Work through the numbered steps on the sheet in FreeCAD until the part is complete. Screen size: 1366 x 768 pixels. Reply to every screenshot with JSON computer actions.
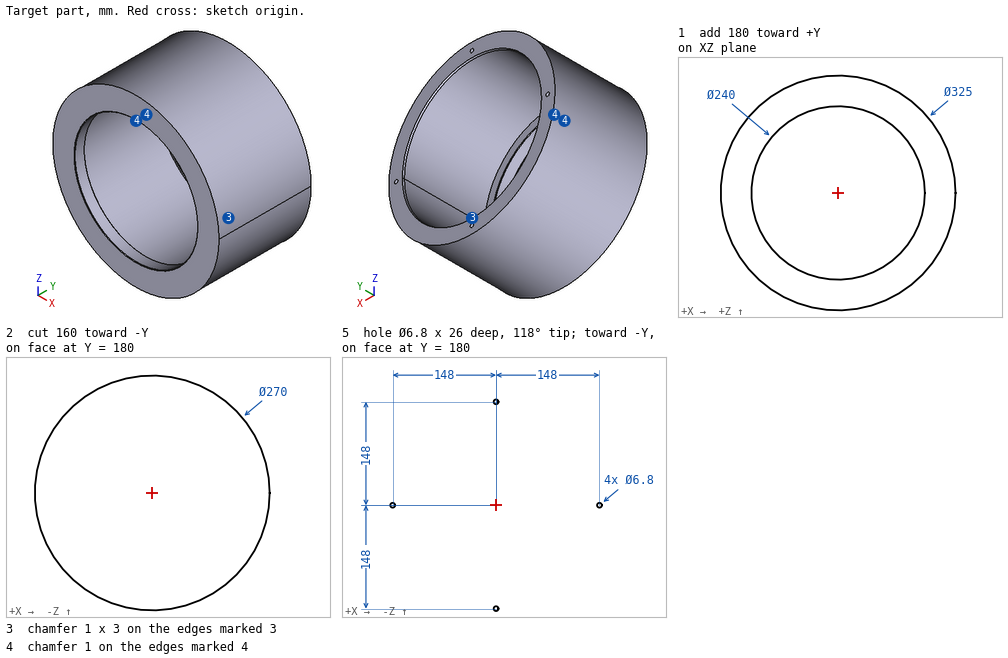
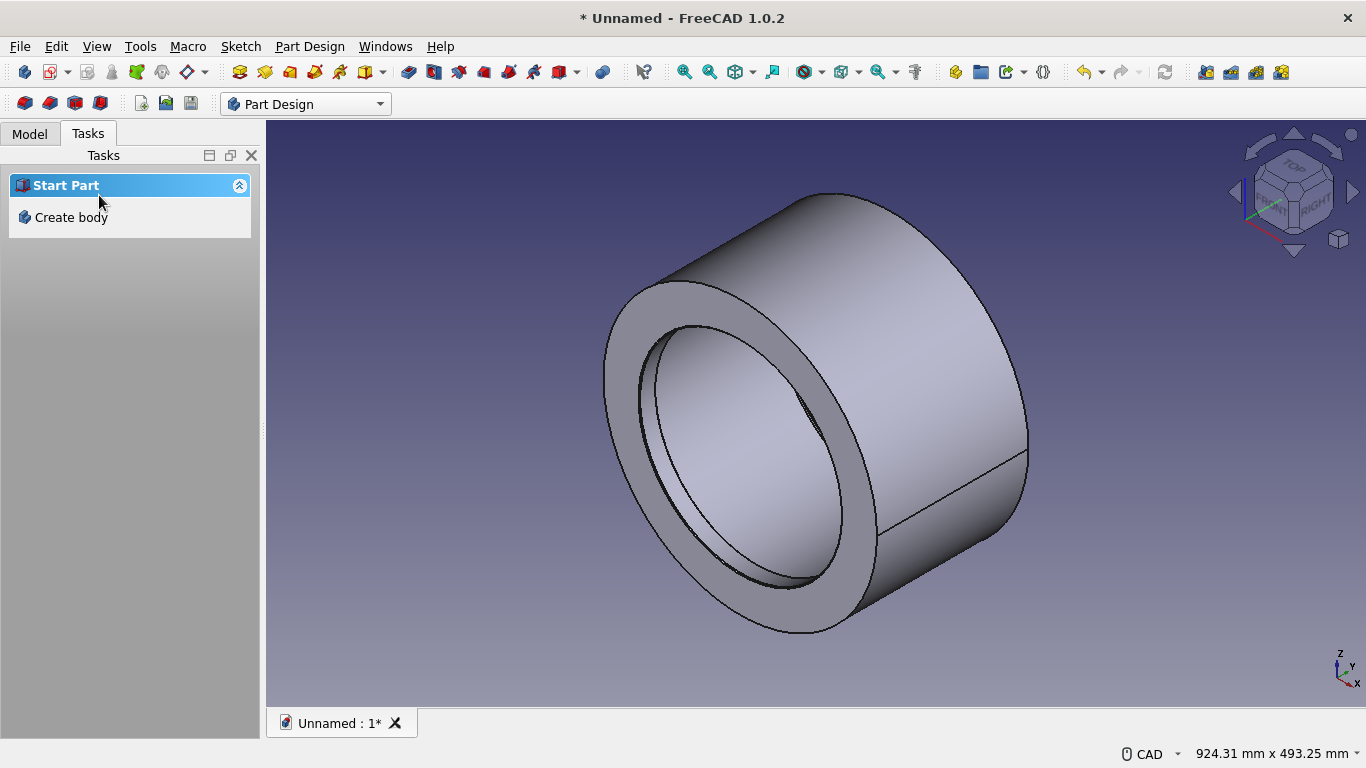
{"action": "key", "text": "4"}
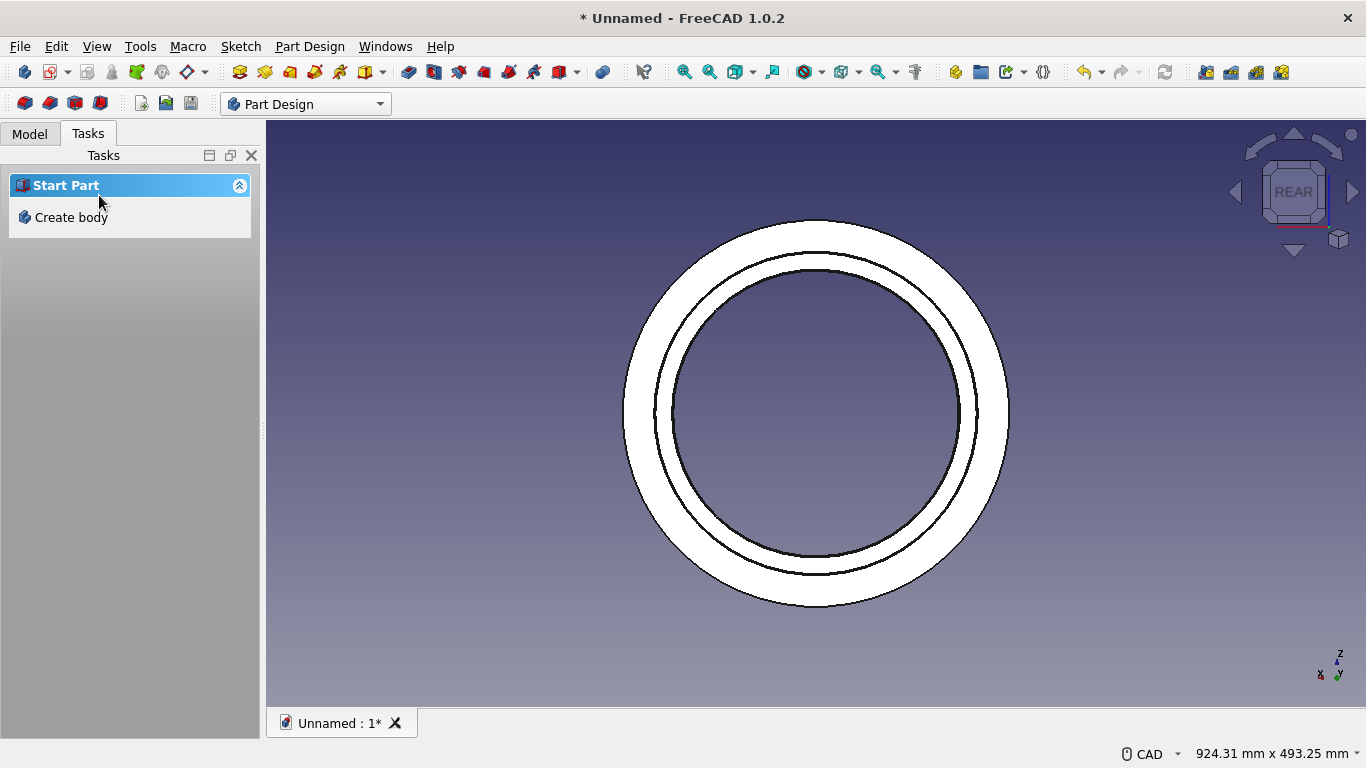
{"action": "left_click", "coordinate": [761, 578]}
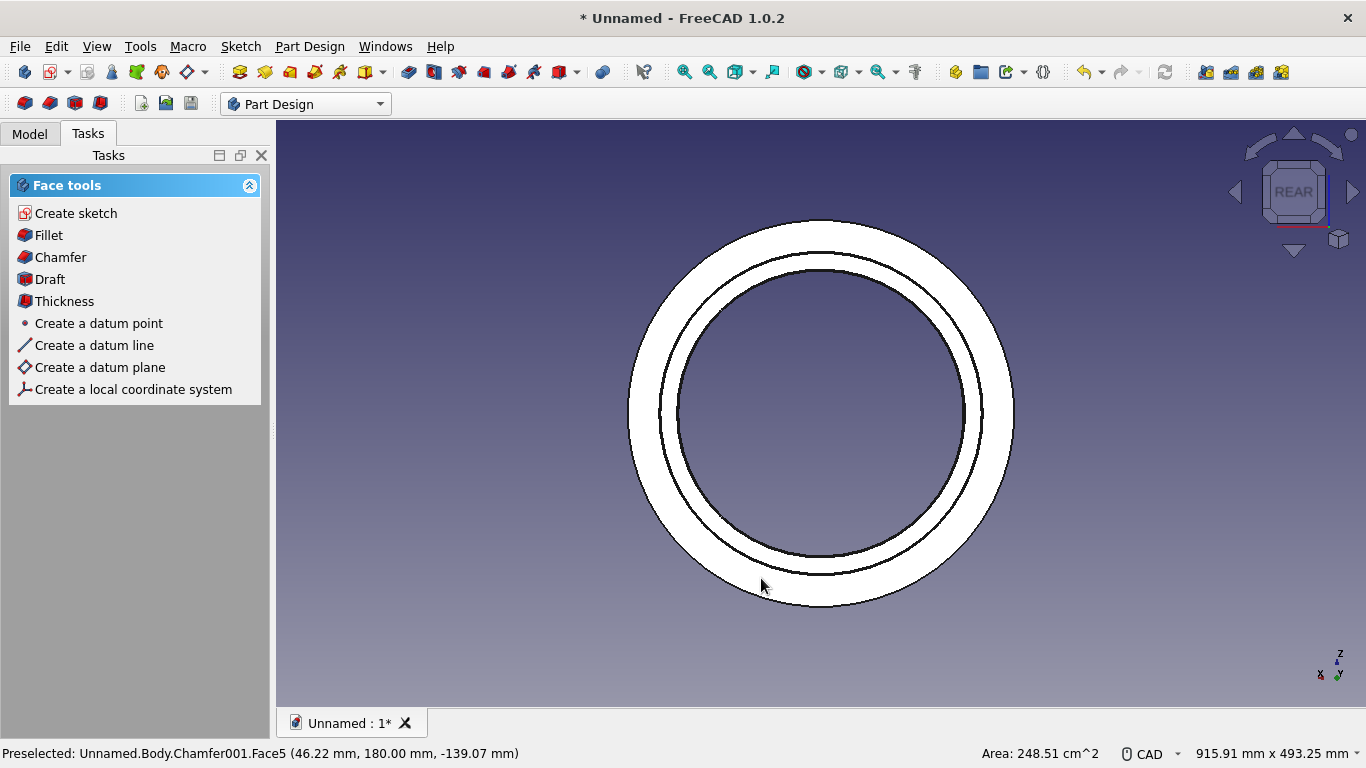
{"action": "left_click", "coordinate": [50, 72]}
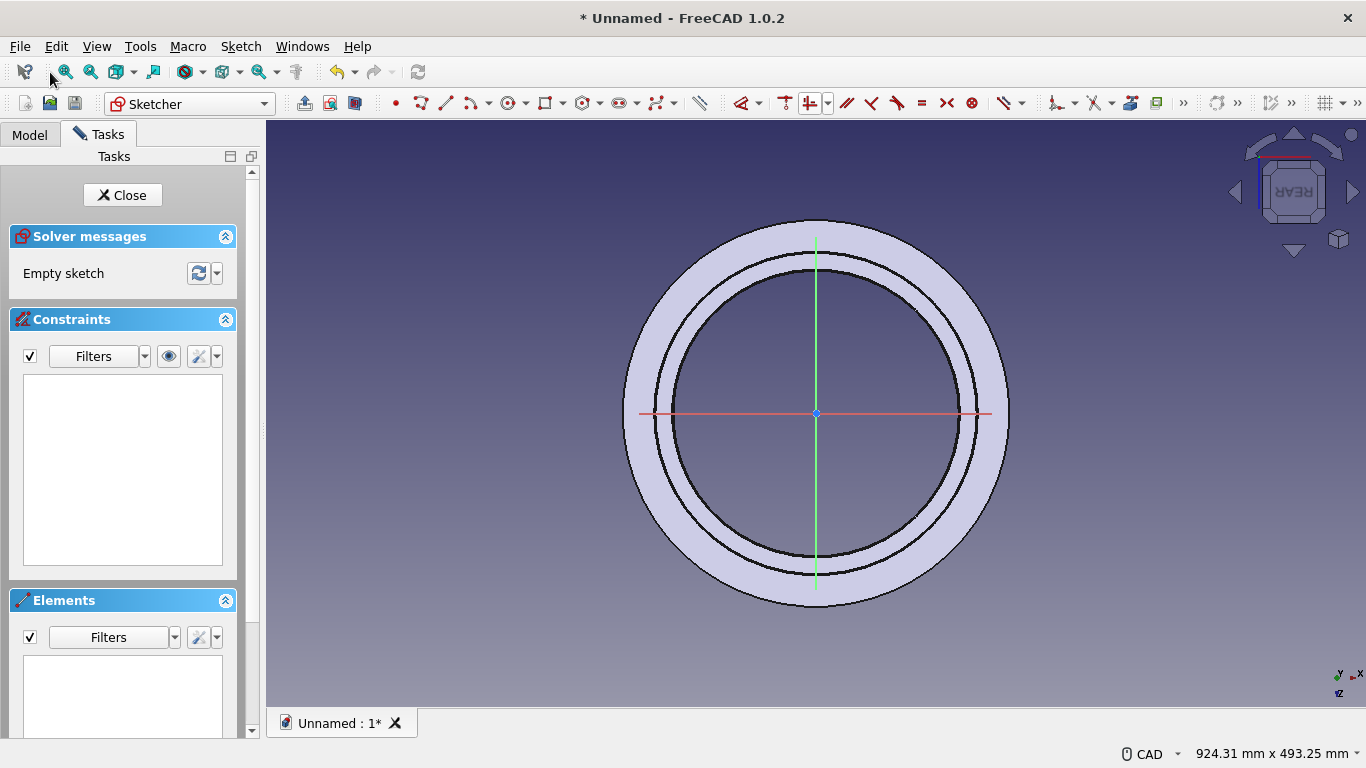
{"action": "left_click", "coordinate": [508, 104]}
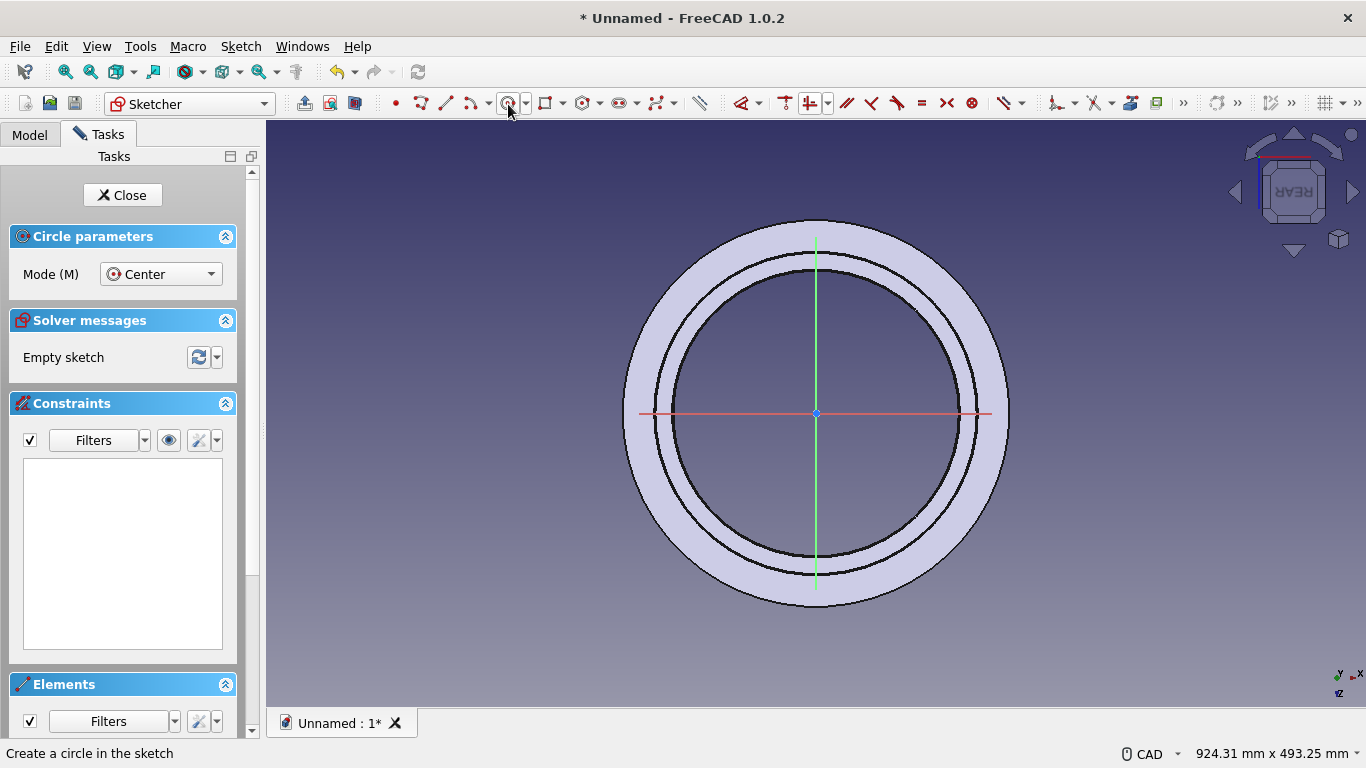
{"action": "scroll", "coordinate": [992, 413], "scroll_direction": "up", "scroll_amount": 9}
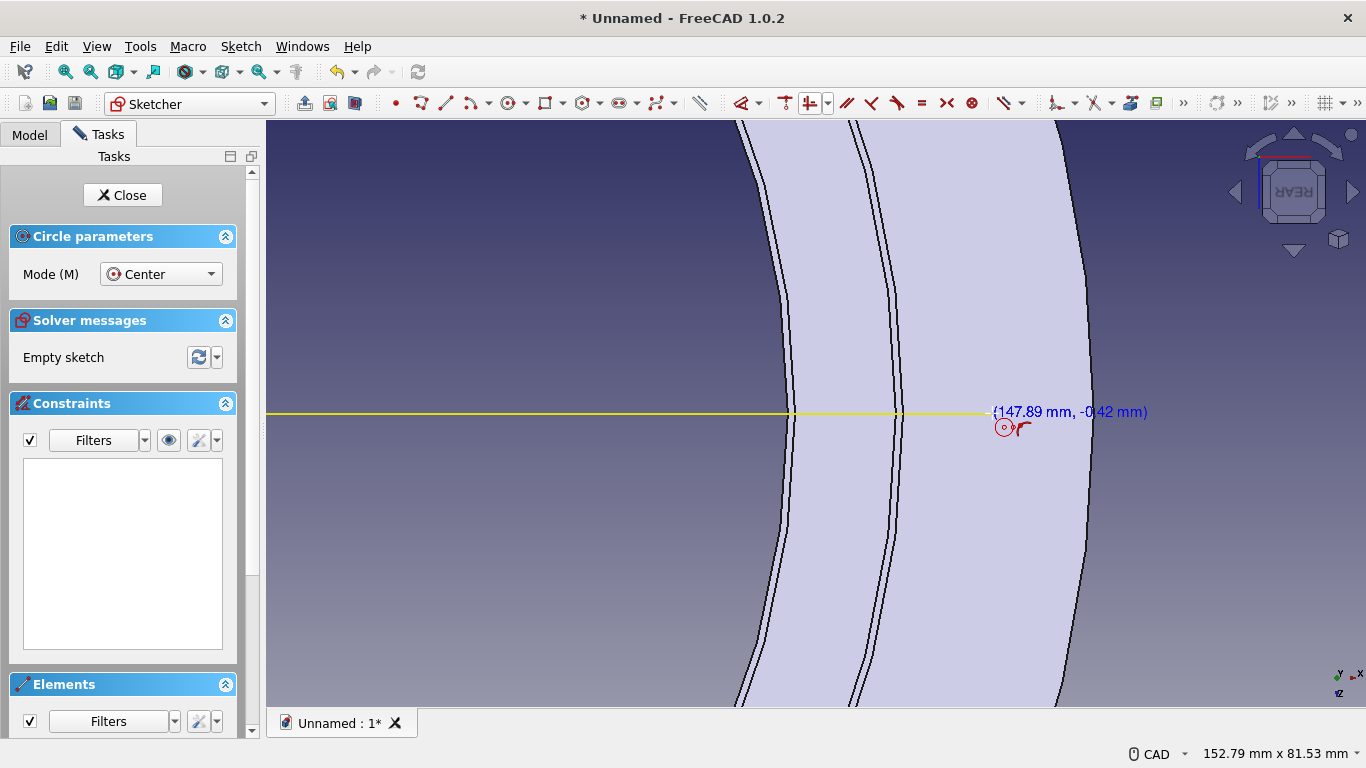
{"action": "scroll", "coordinate": [911, 414], "scroll_direction": "down", "scroll_amount": 9}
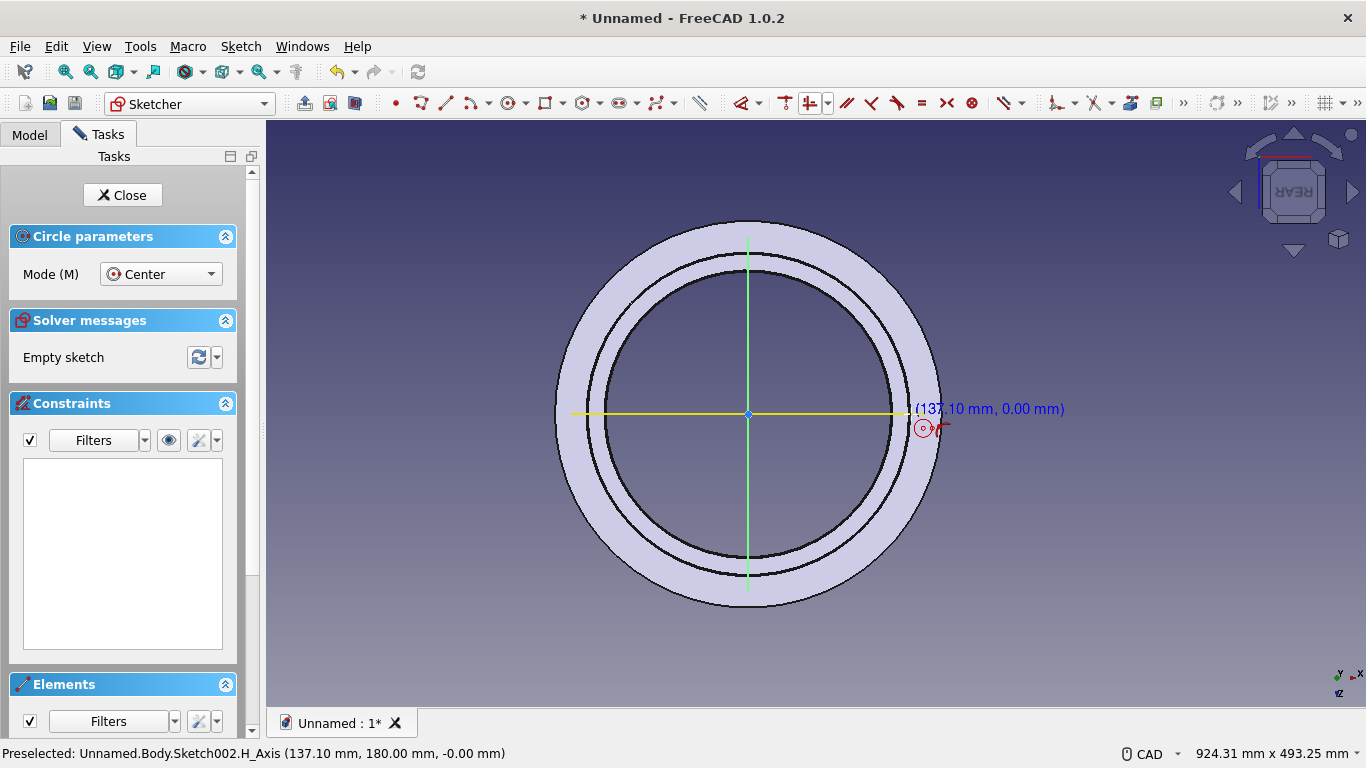
{"action": "left_click", "coordinate": [924, 414]}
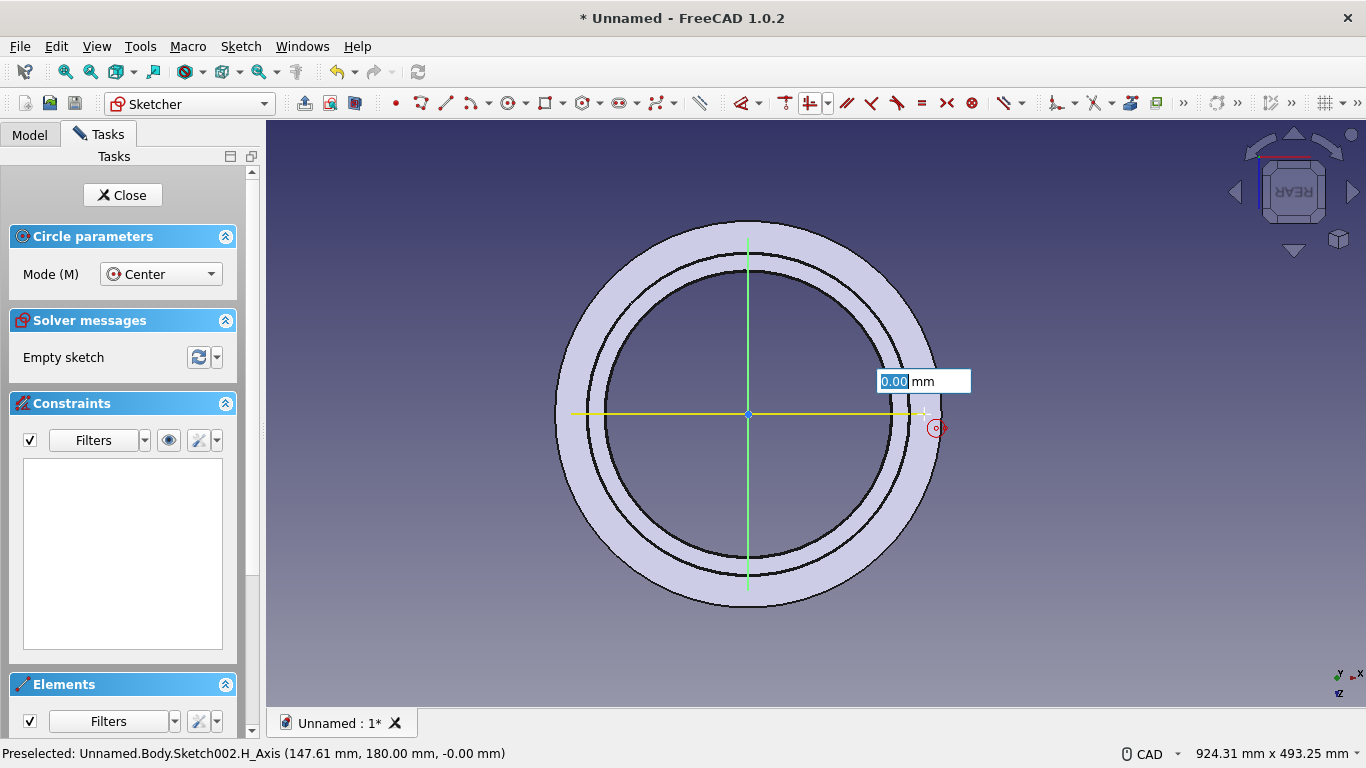
{"action": "scroll", "coordinate": [923, 418], "scroll_direction": "up", "scroll_amount": 8}
{"action": "mouse_move", "coordinate": [921, 417]}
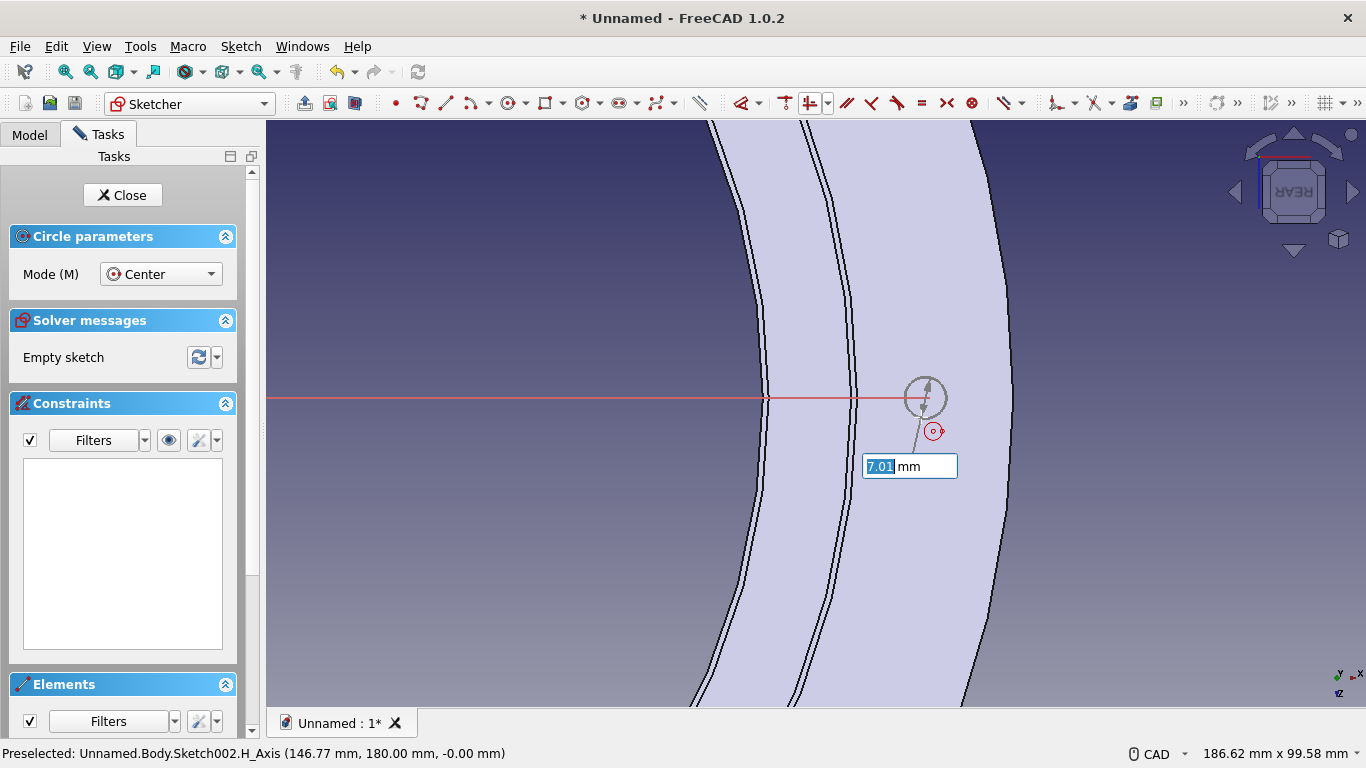
{"action": "type", "text": "6.8"}
{"action": "key", "text": "Return"}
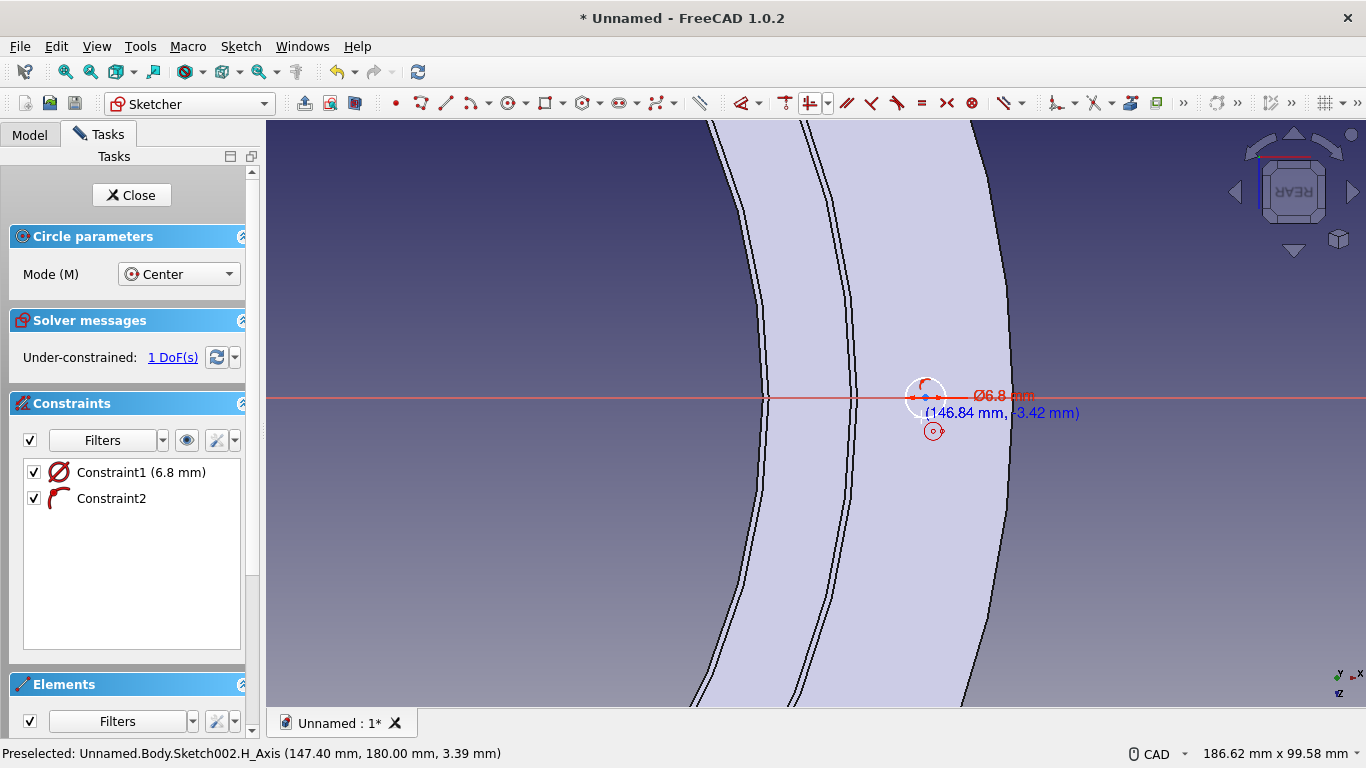
{"action": "scroll", "coordinate": [923, 417], "scroll_direction": "down", "scroll_amount": 8}